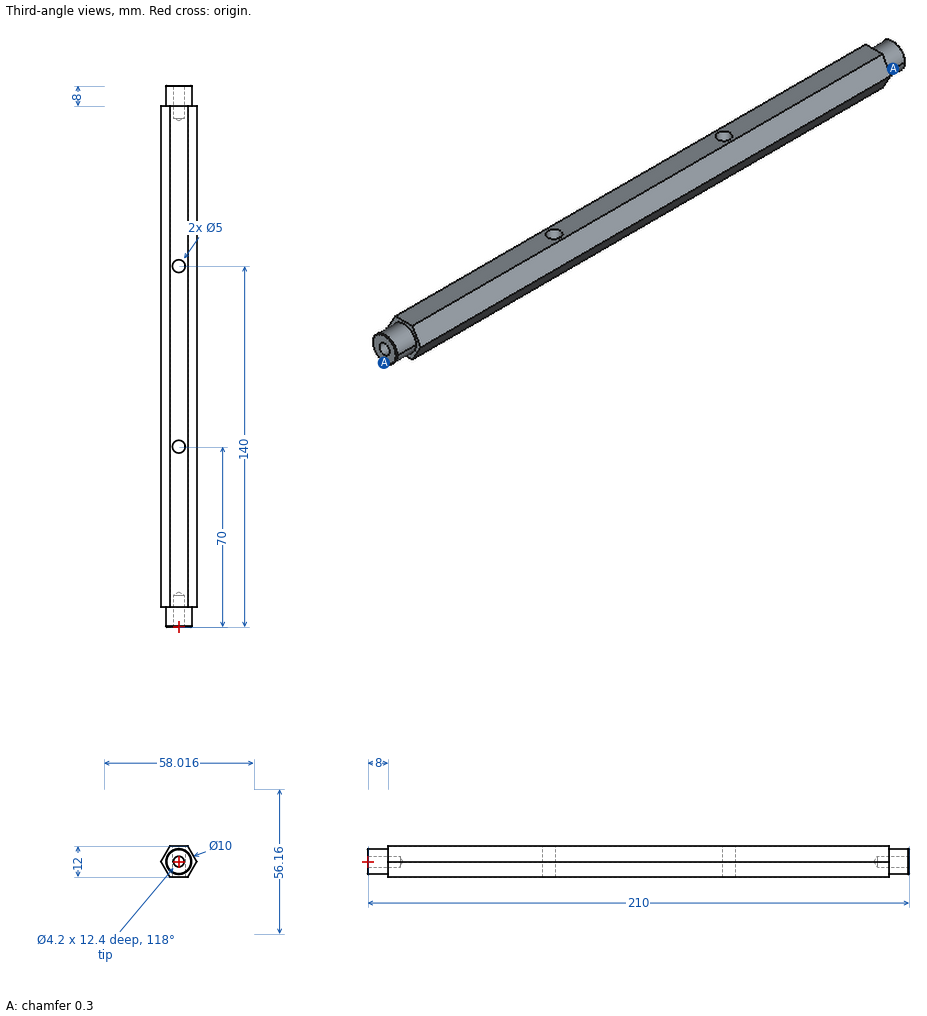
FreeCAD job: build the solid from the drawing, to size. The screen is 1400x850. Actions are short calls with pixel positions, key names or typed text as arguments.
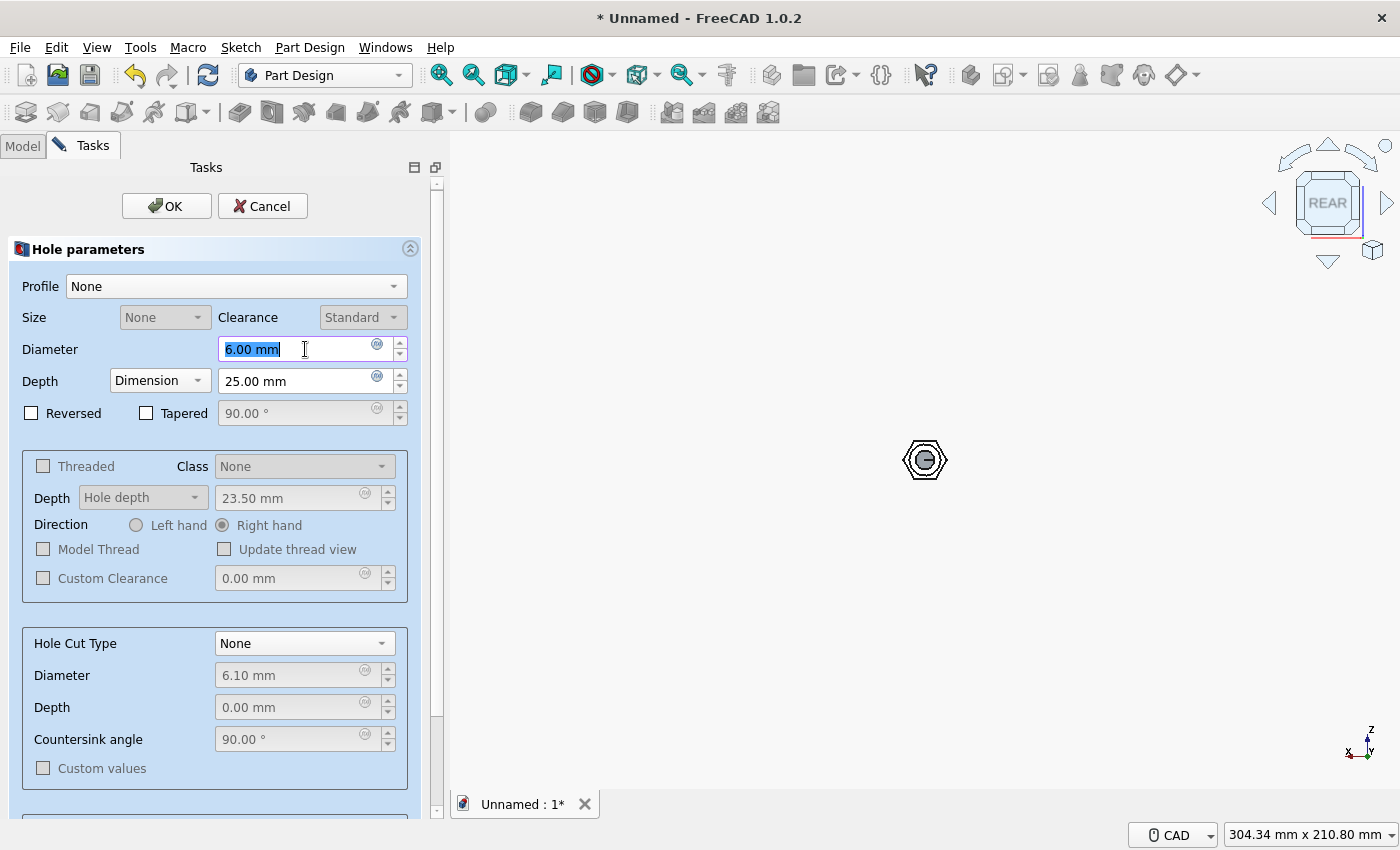
text(4.2)
key(Tab)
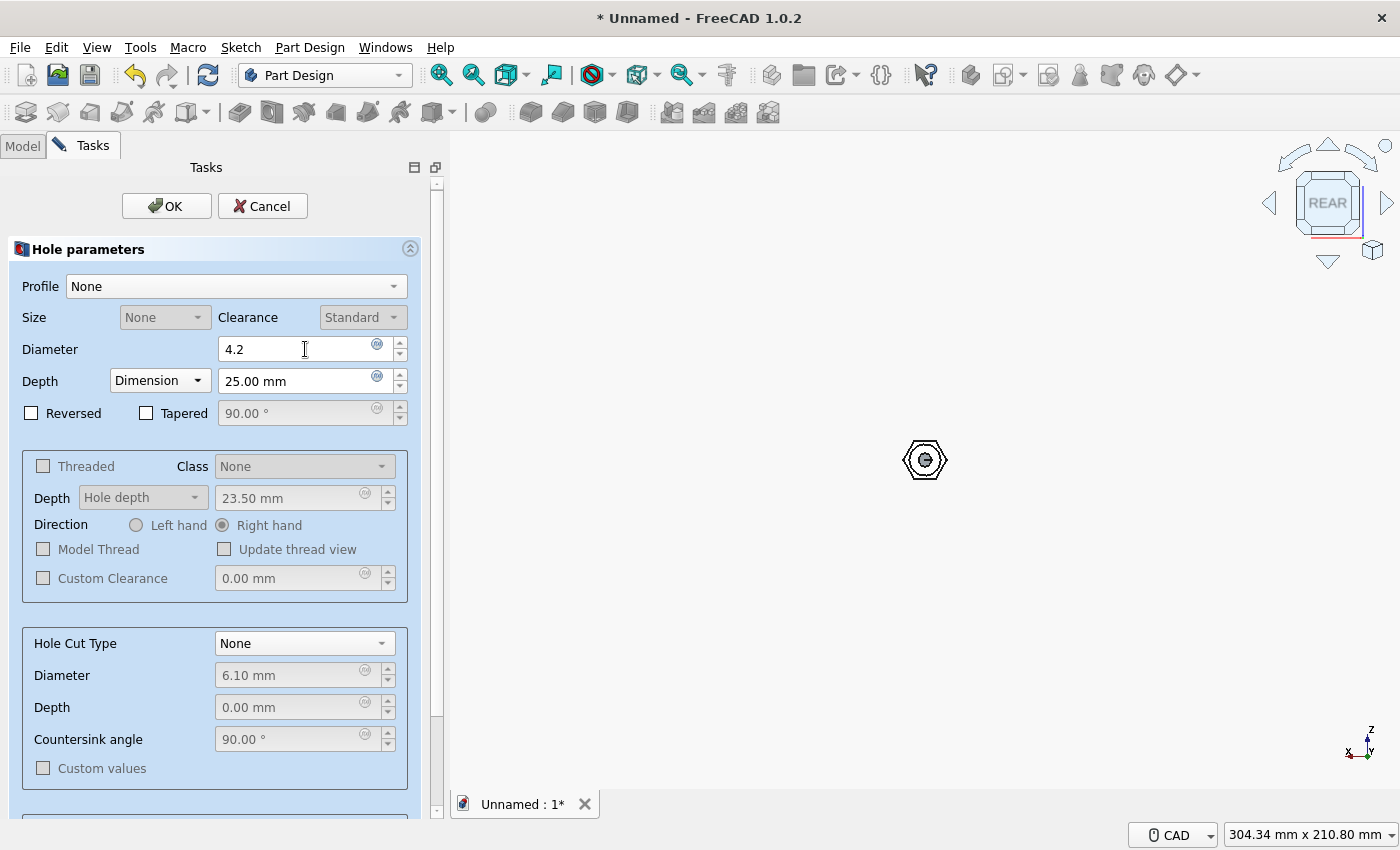
triple_click(305, 381)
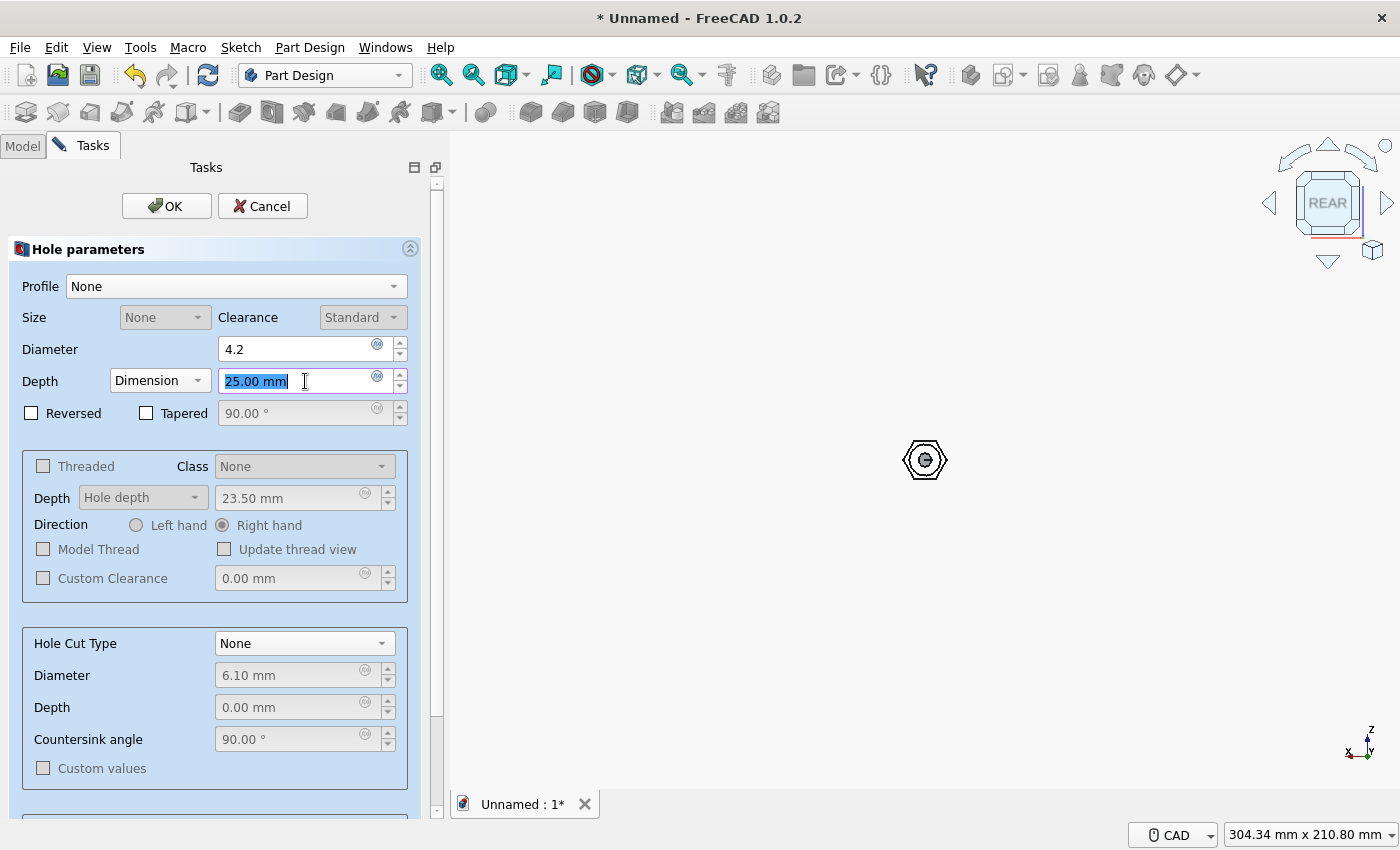
text(12.4)
key(Tab)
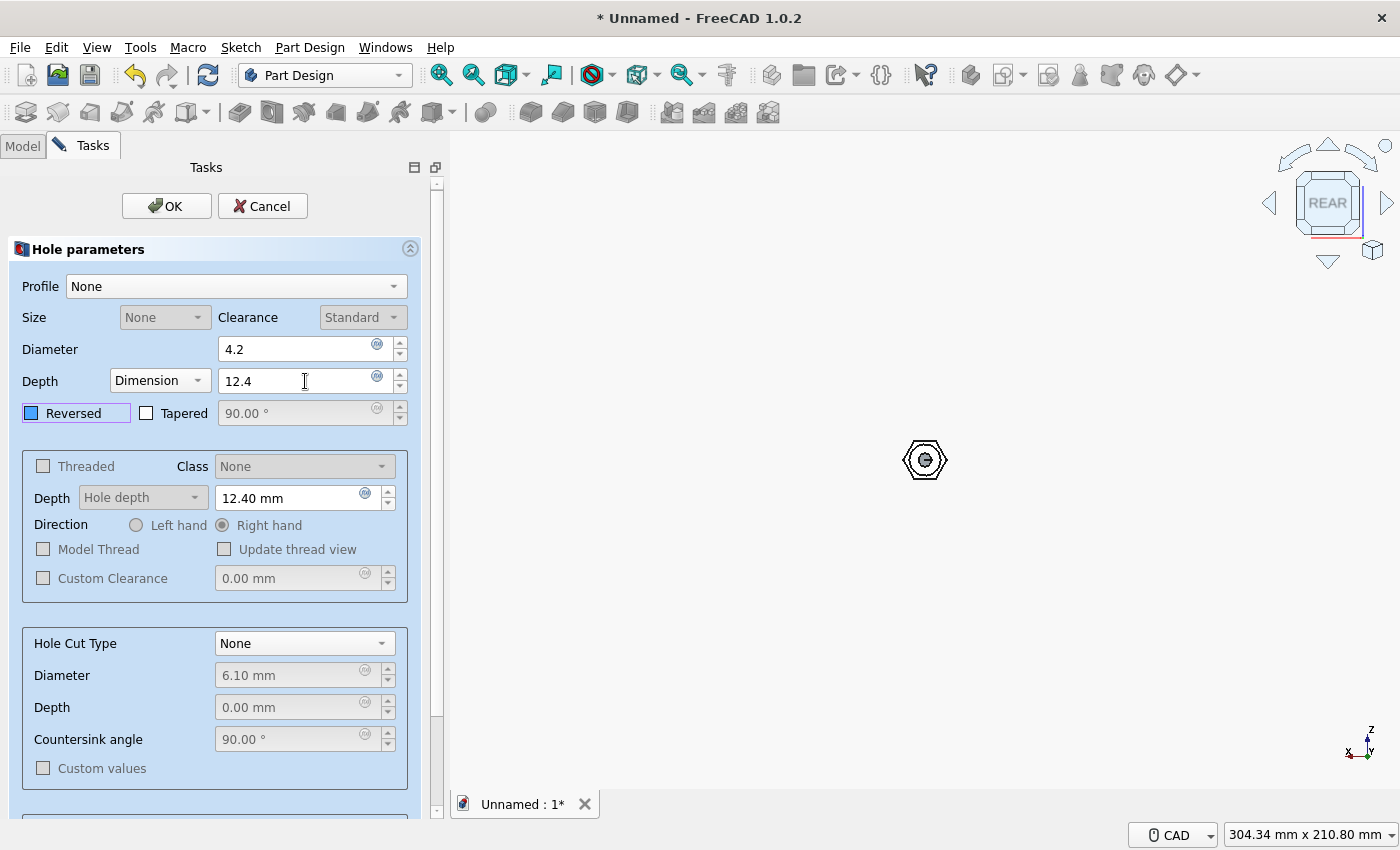
click(167, 206)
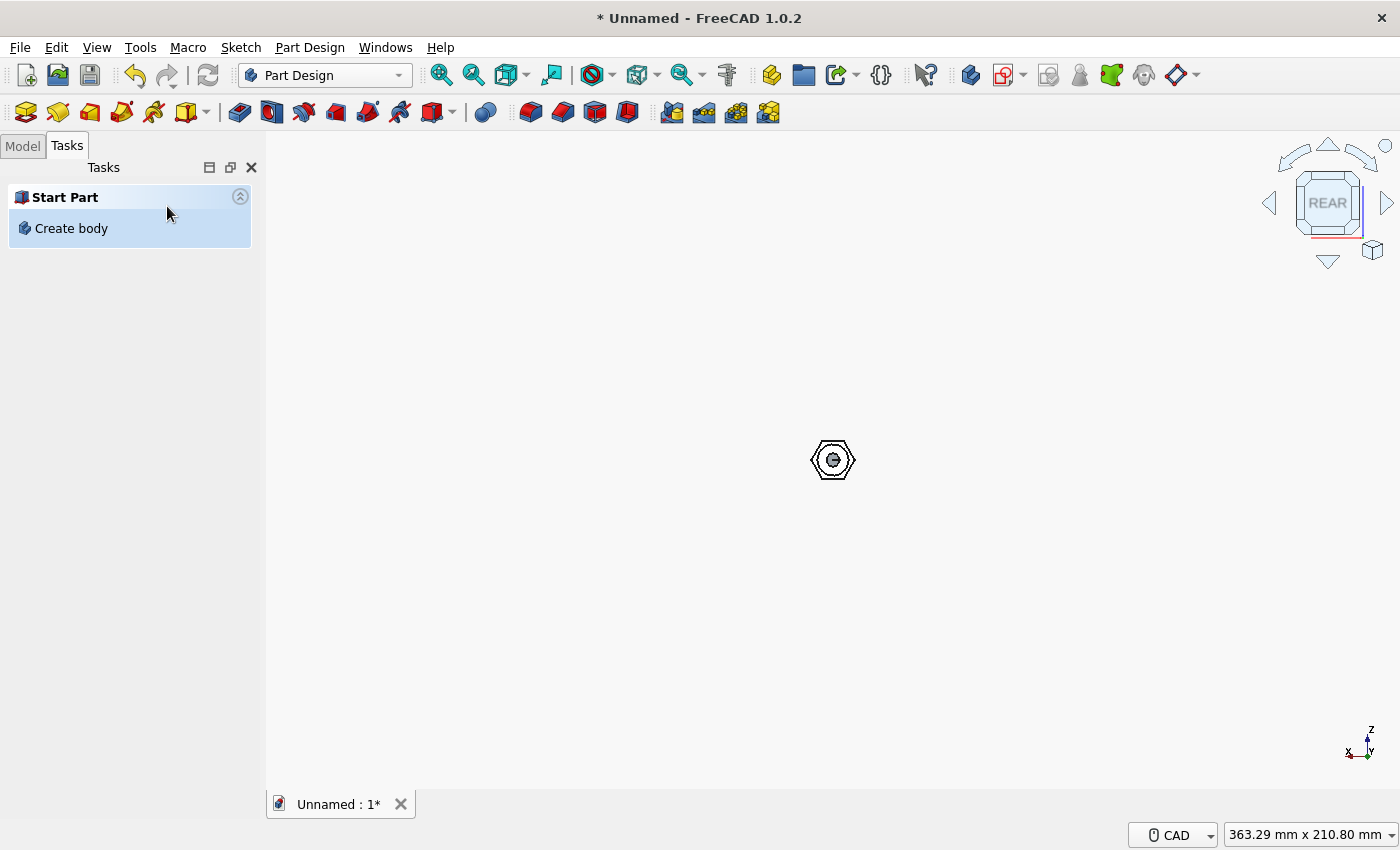
click(442, 76)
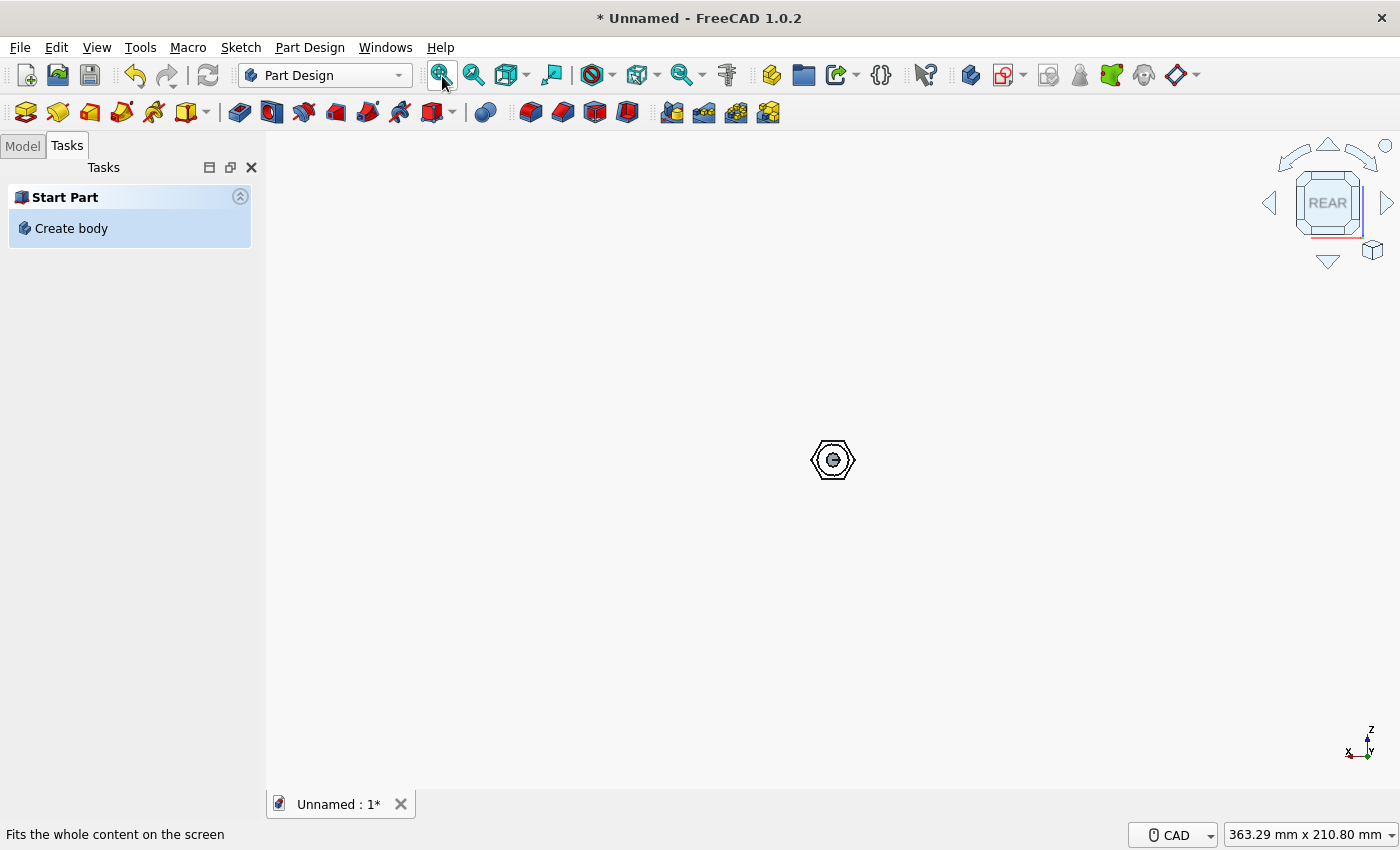
click(849, 459)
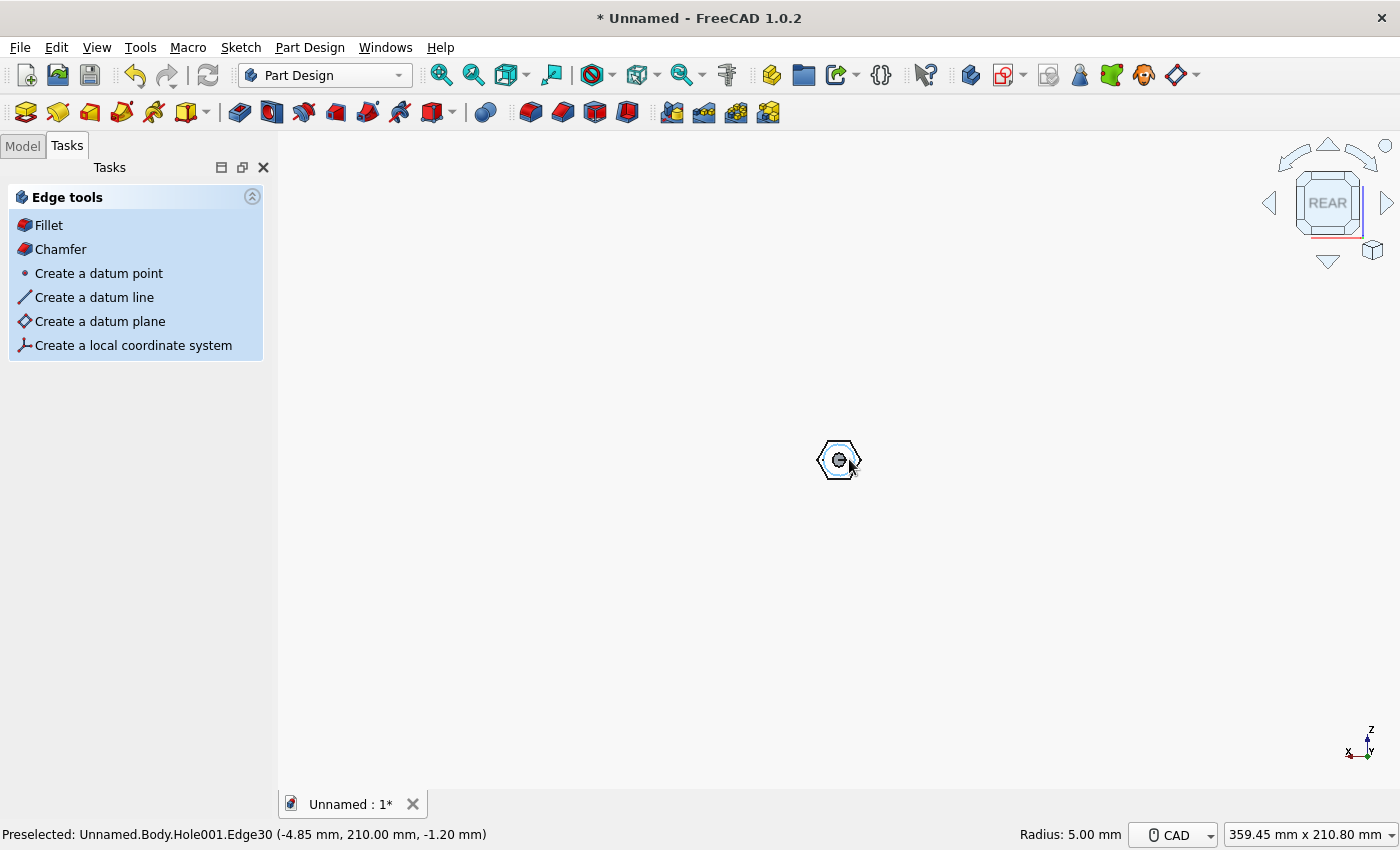
key(0)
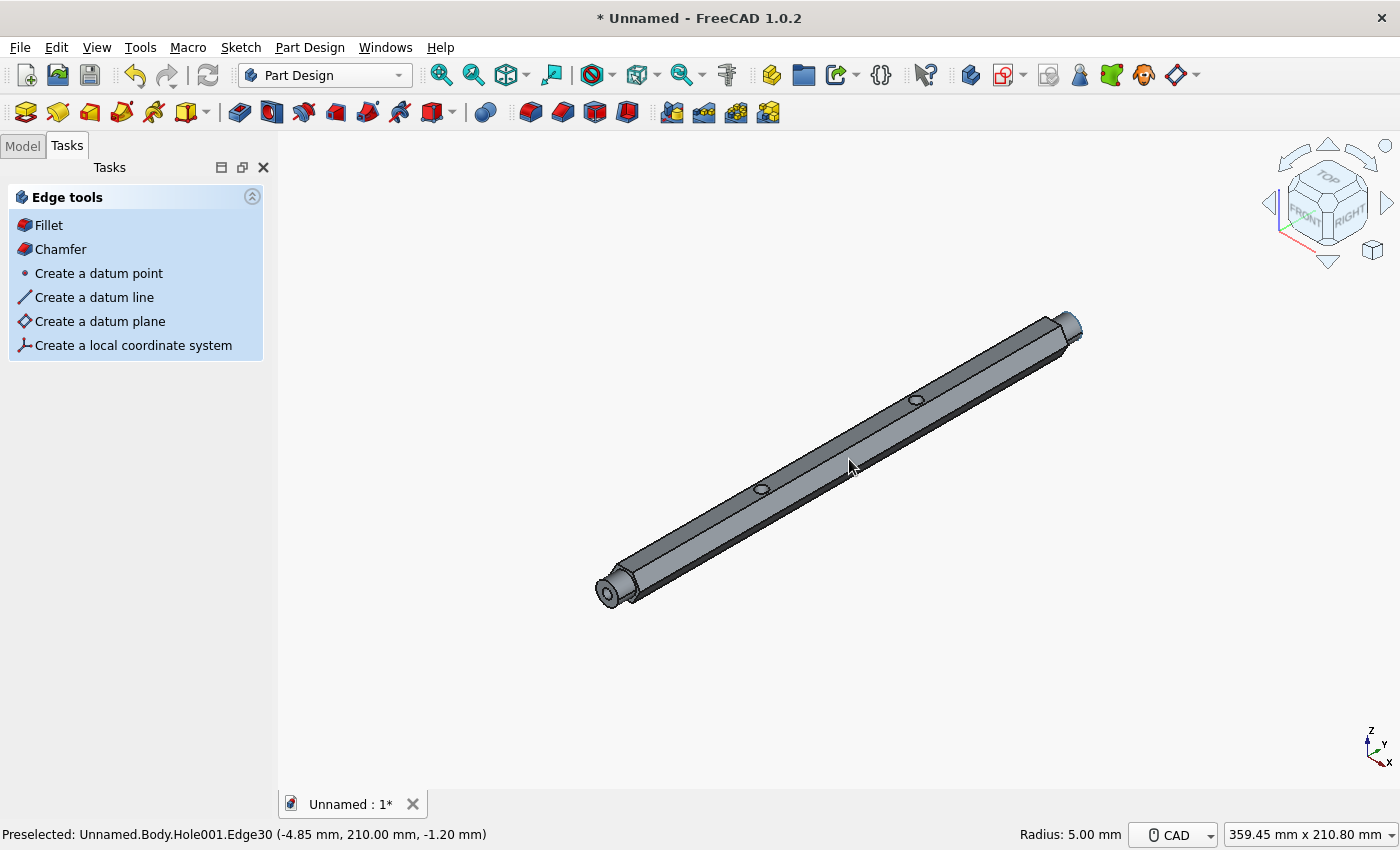
click(596, 586, ctrl)